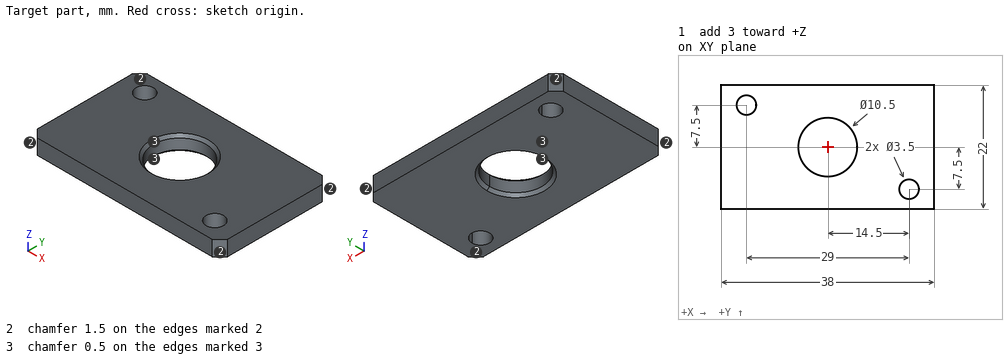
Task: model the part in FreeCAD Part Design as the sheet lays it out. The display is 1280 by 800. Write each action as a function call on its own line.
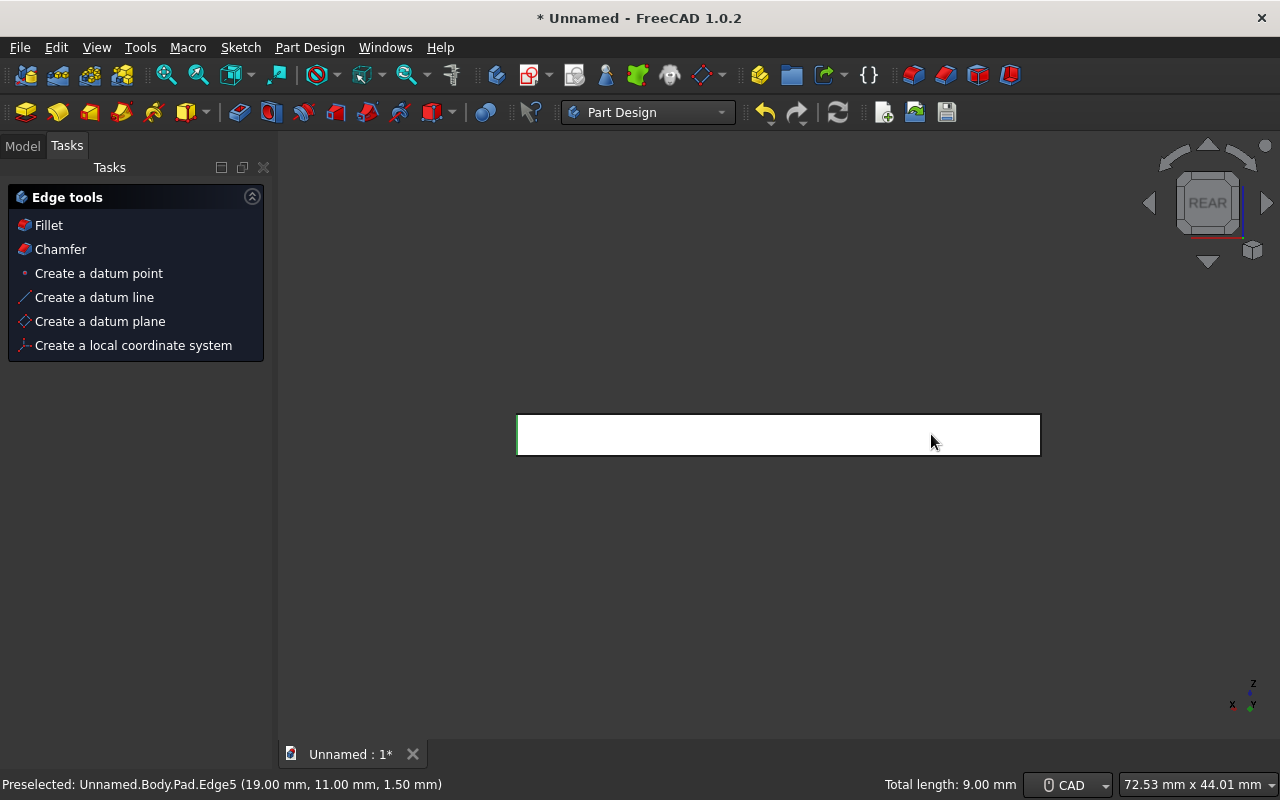
click(1041, 434, ctrl)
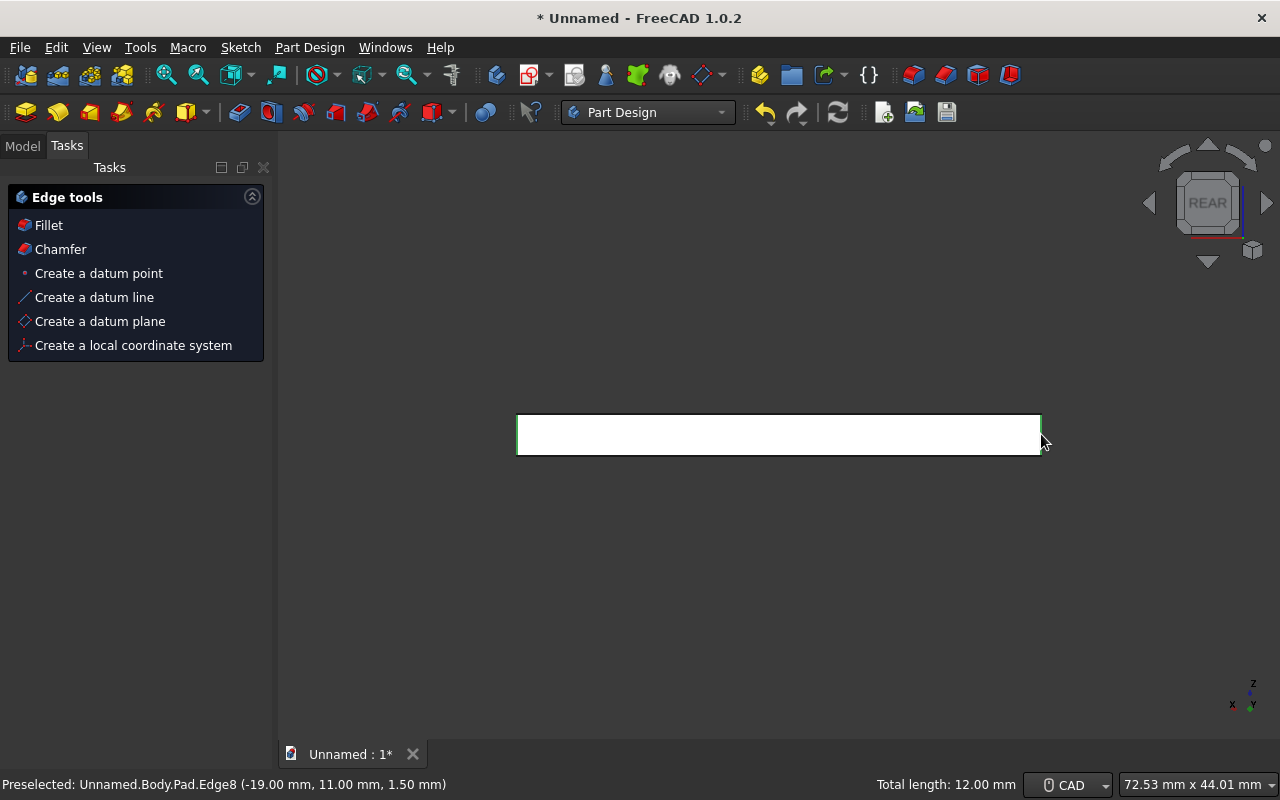
click(946, 76)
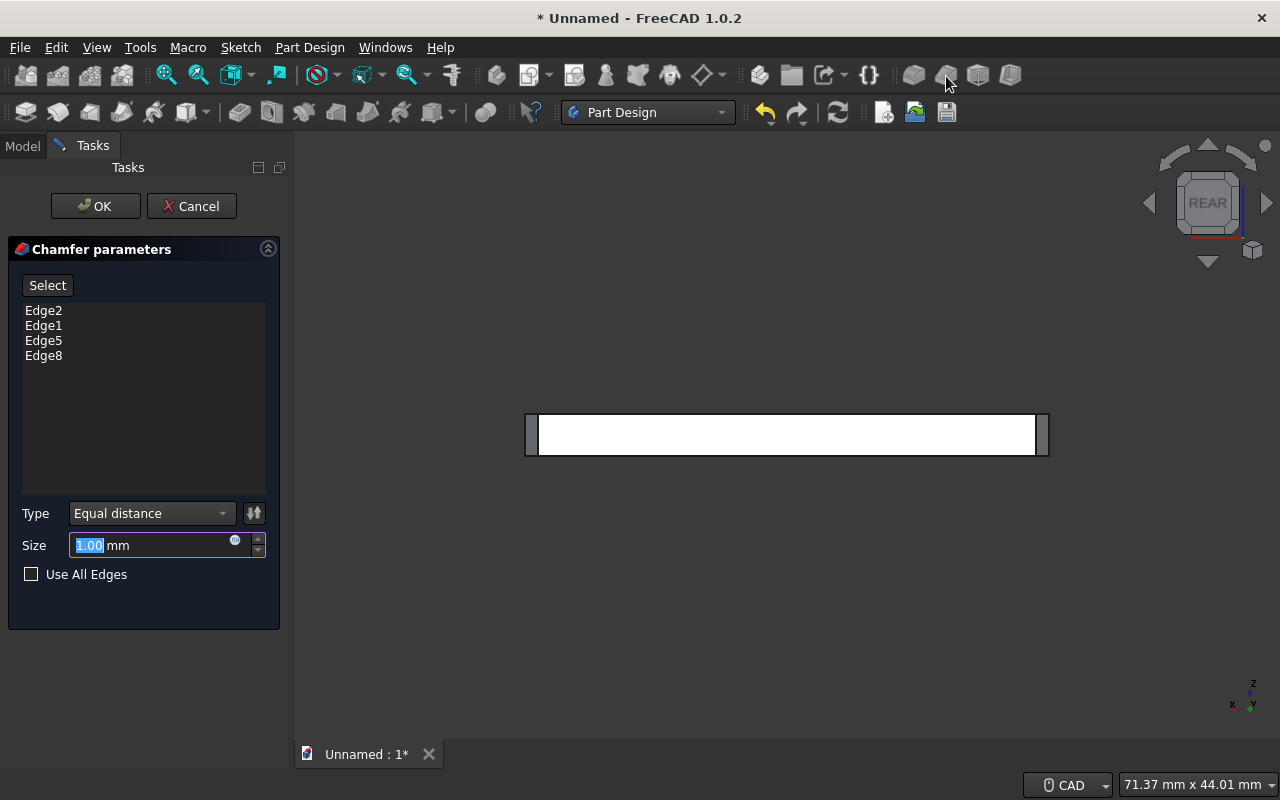
text(1.5)
key(Tab)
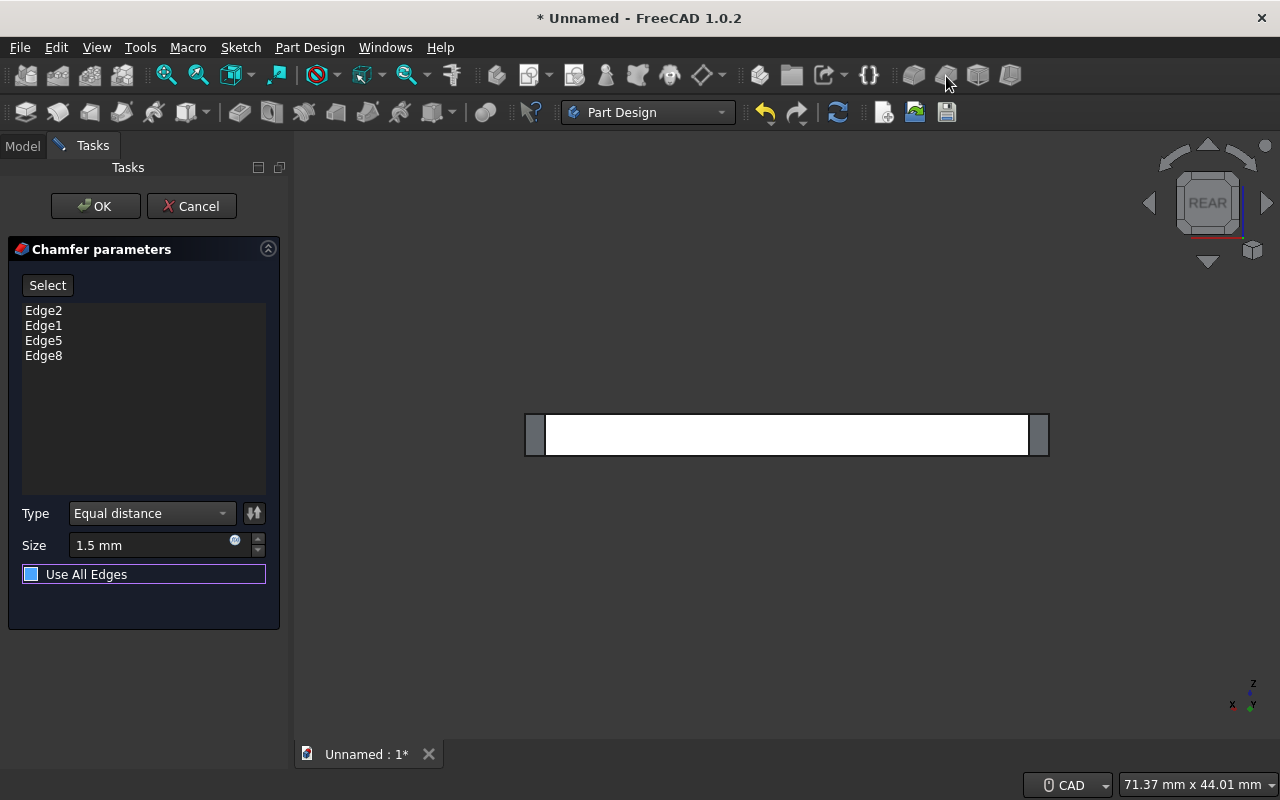
click(96, 206)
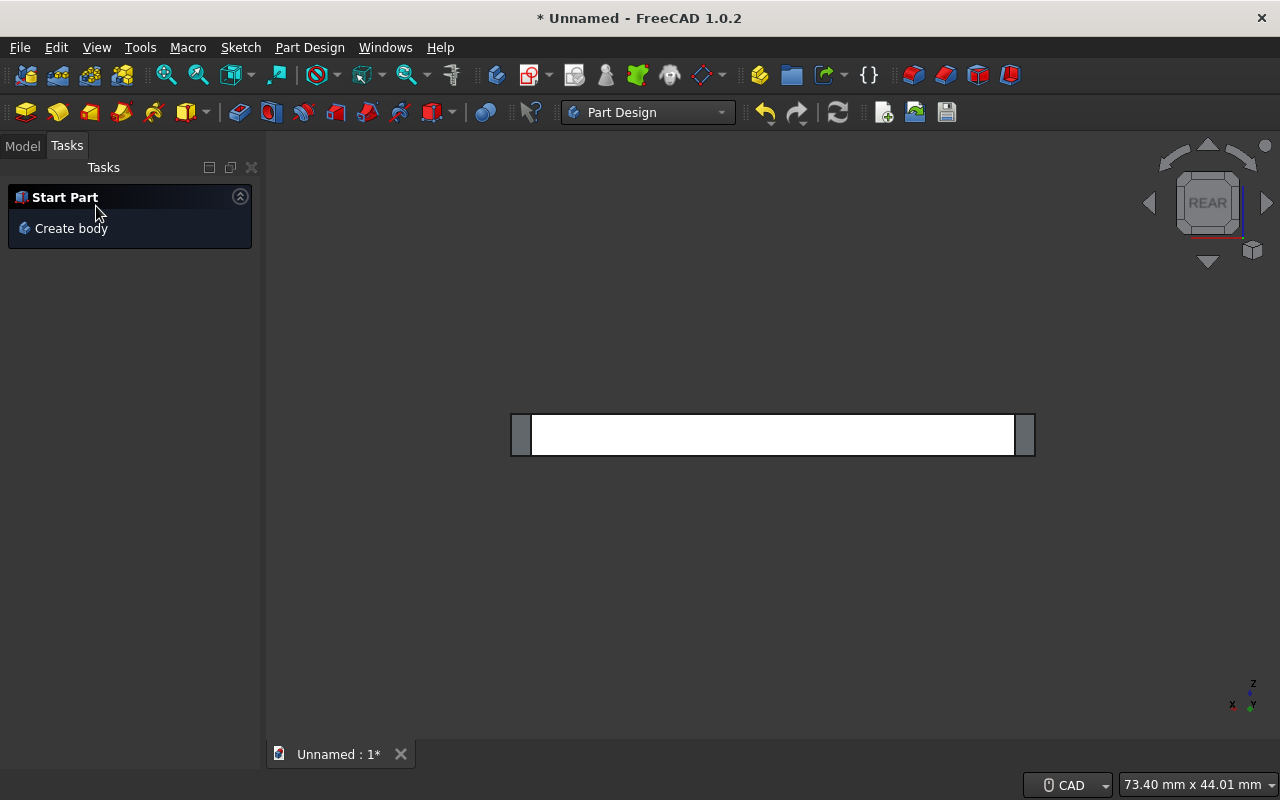
key(0)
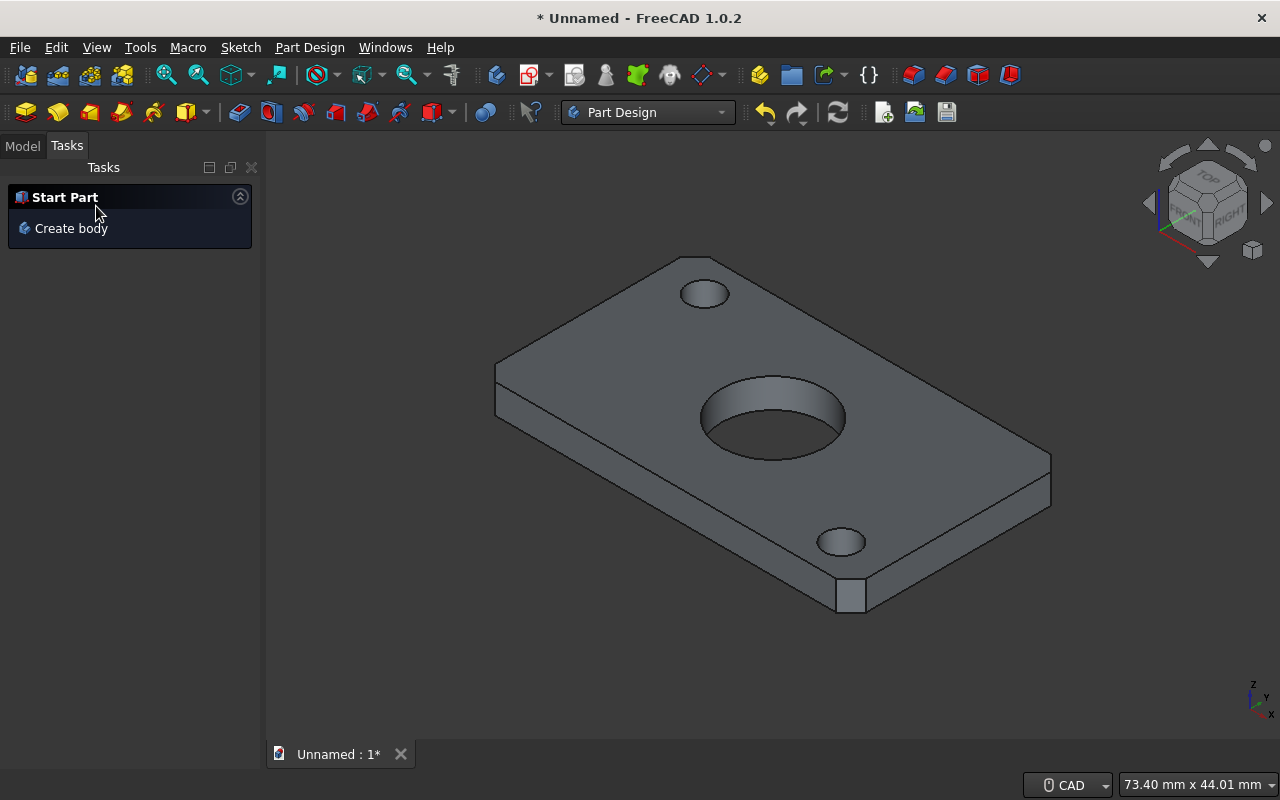
click(722, 387)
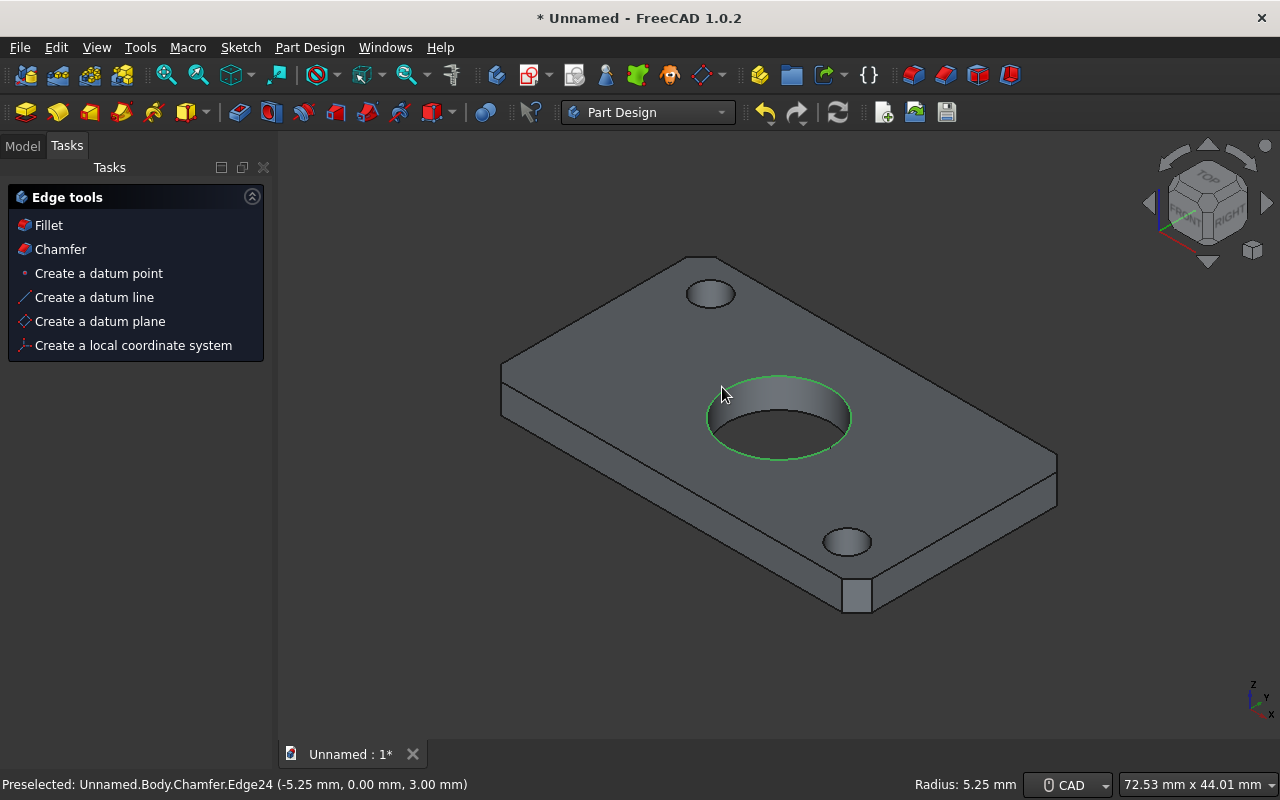
key(2)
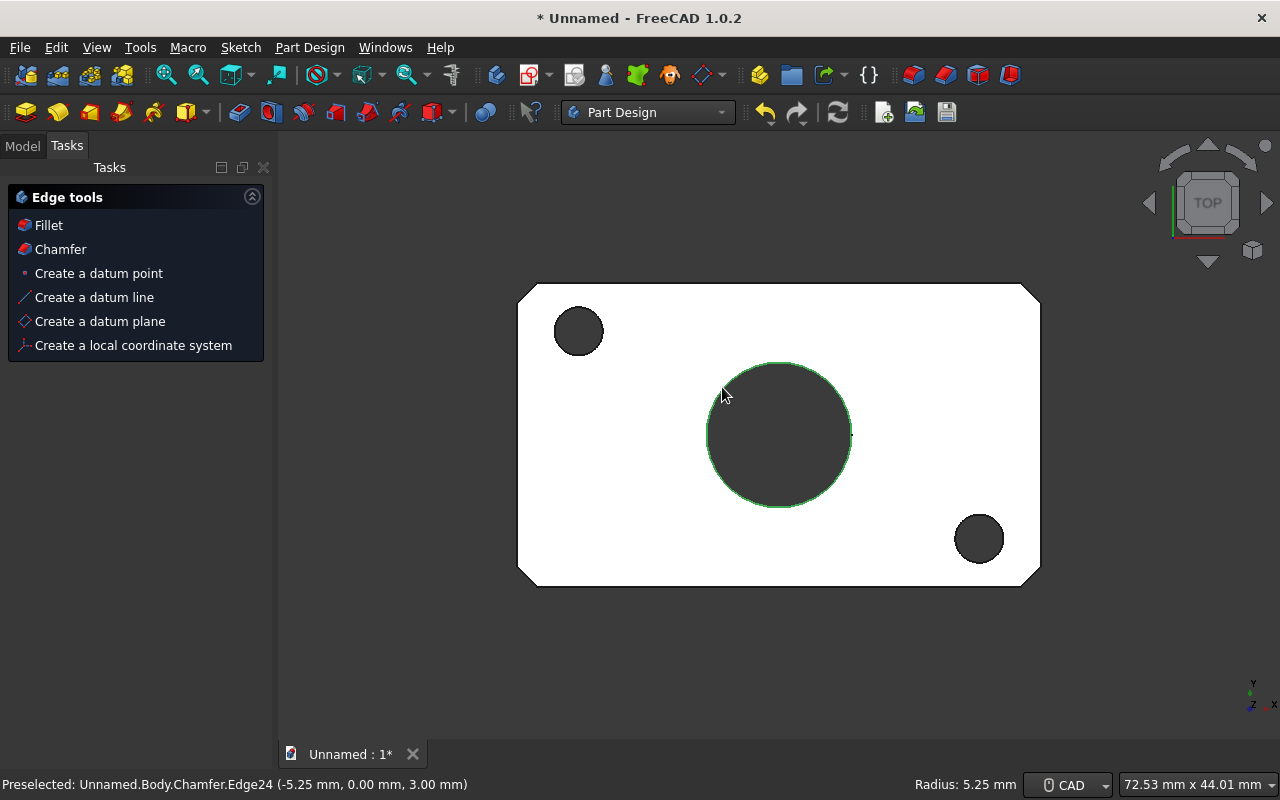
key(1)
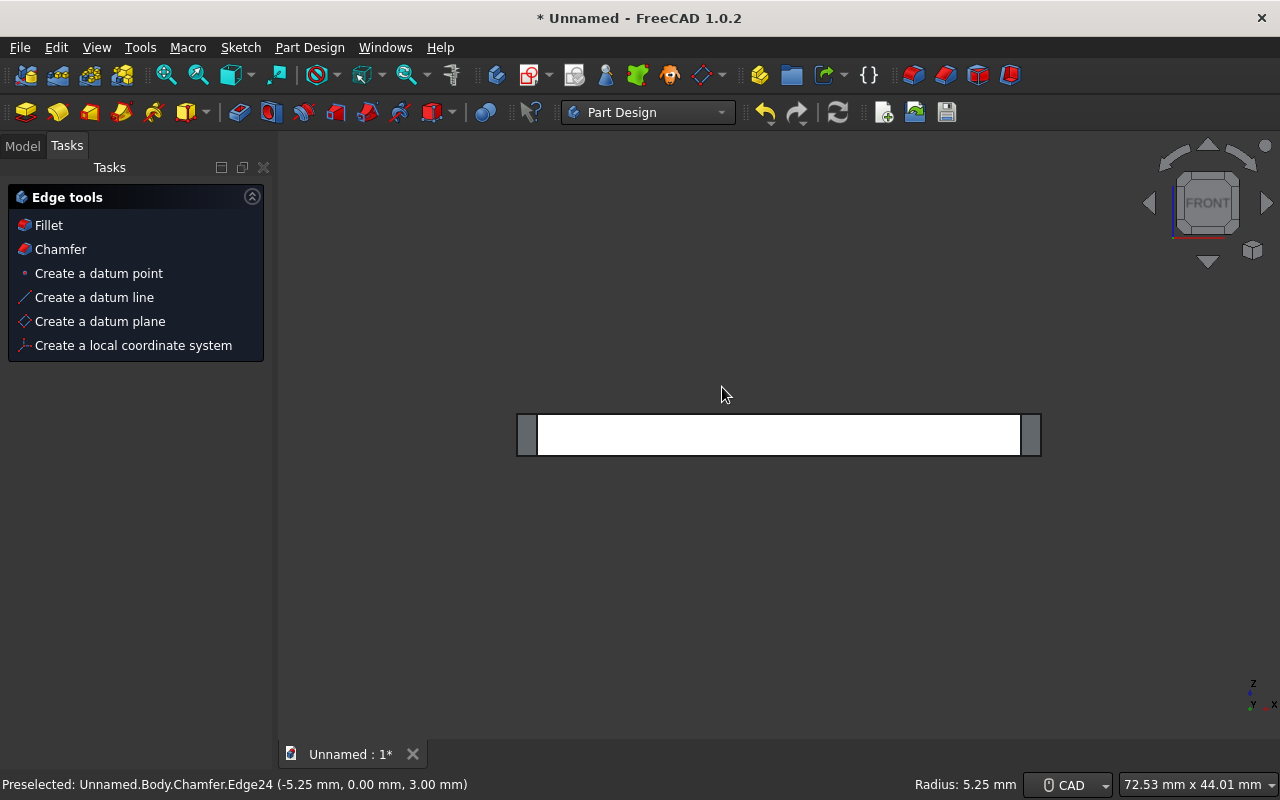
key(3)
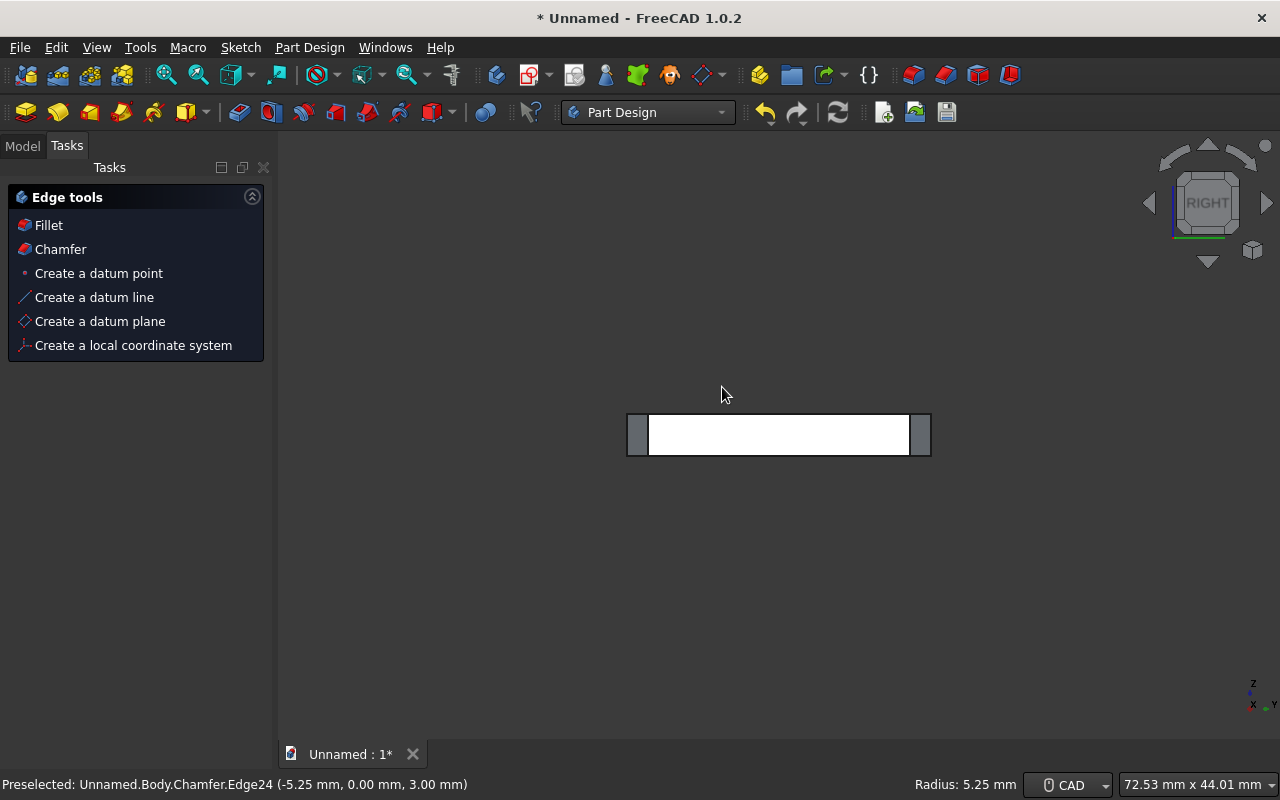
key(v)
key(f)